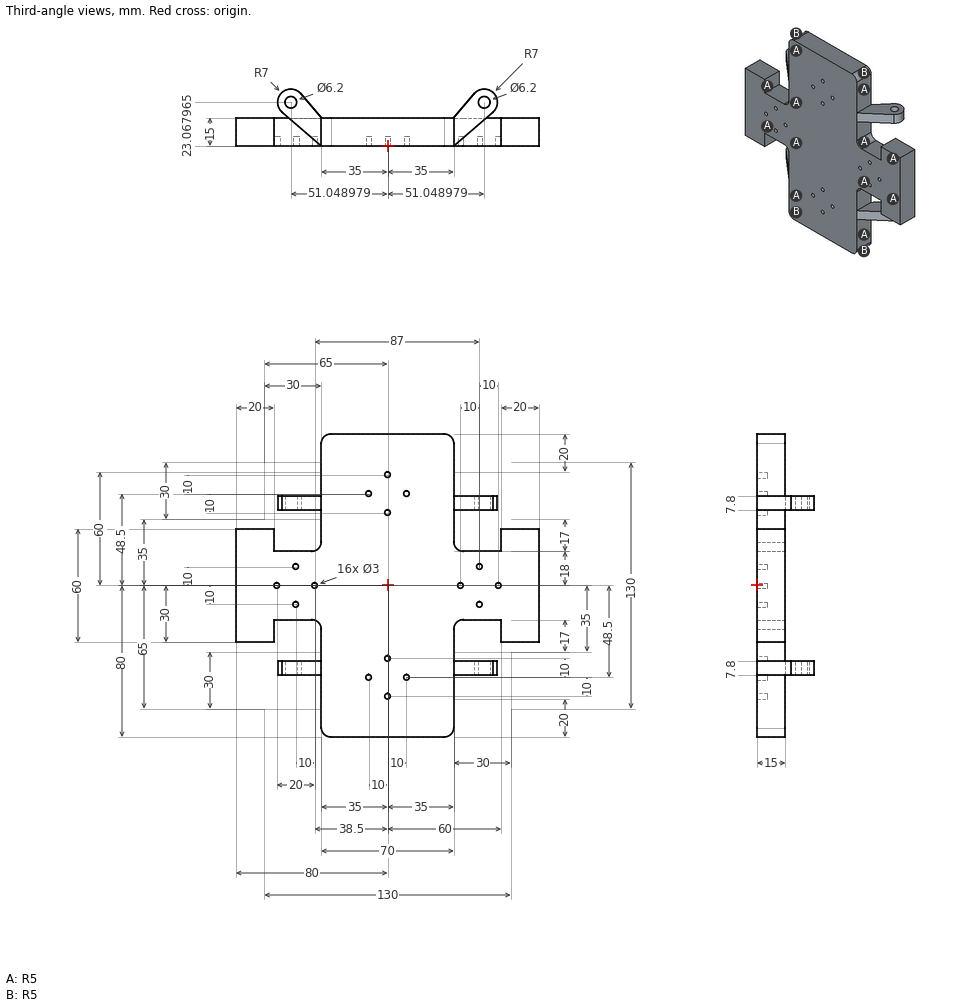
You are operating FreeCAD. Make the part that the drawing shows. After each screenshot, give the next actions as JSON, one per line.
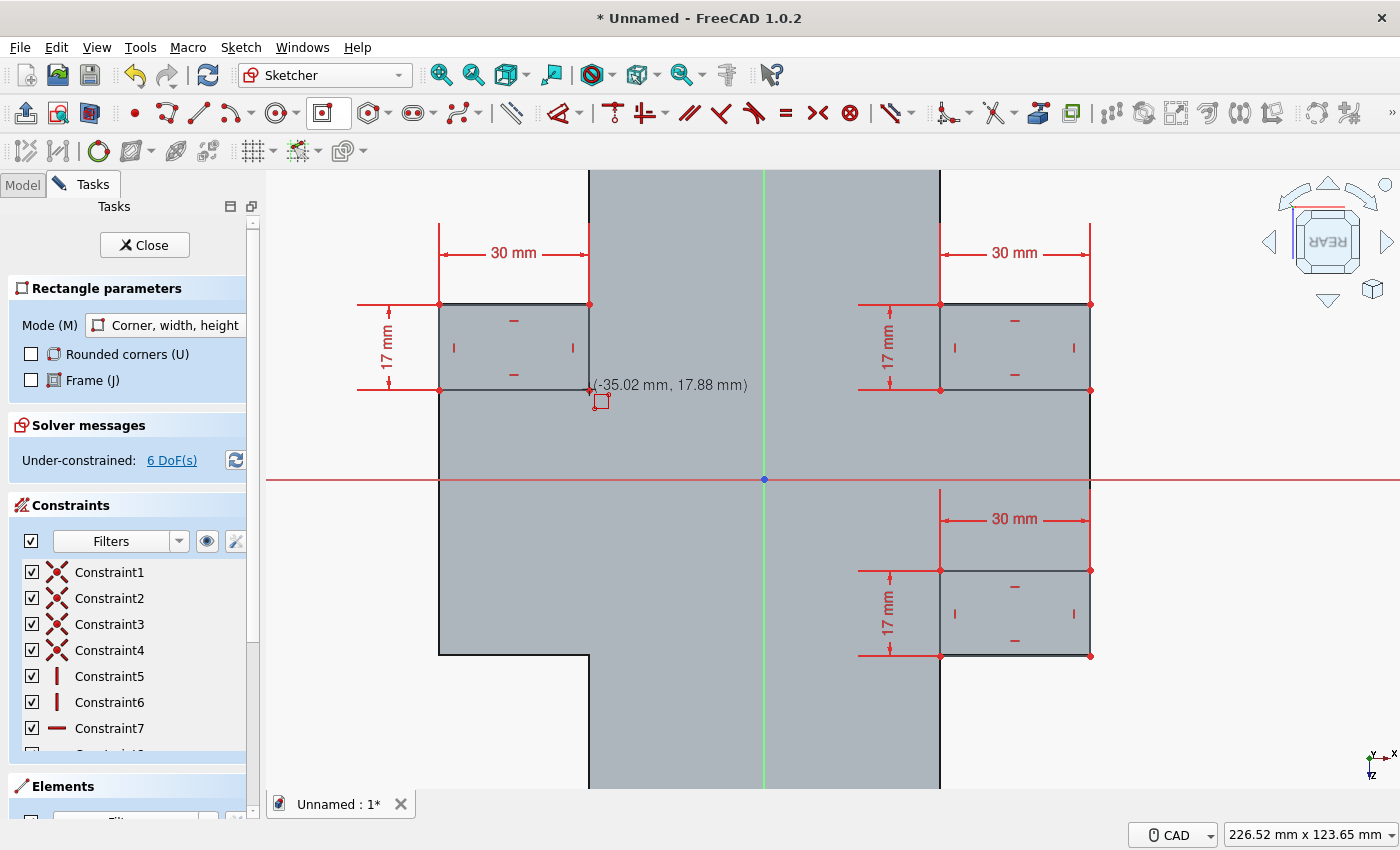
{"action": "left_click", "coordinate": [439, 570]}
{"action": "mouse_move", "coordinate": [589, 655]}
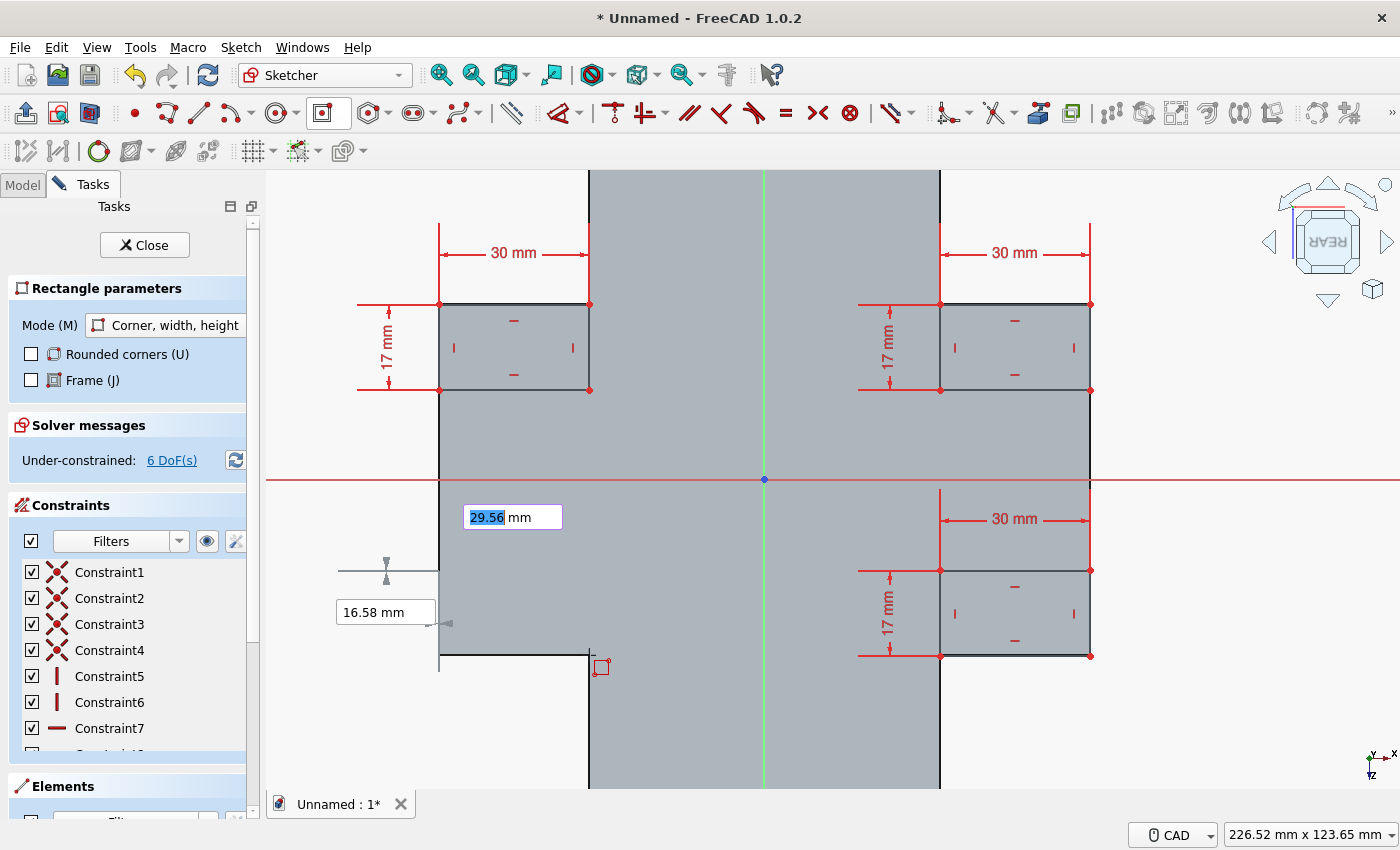
{"action": "type", "text": "30"}
{"action": "key", "text": "Tab"}
{"action": "type", "text": "17"}
{"action": "key", "text": "Return"}
{"action": "key", "text": "Escape"}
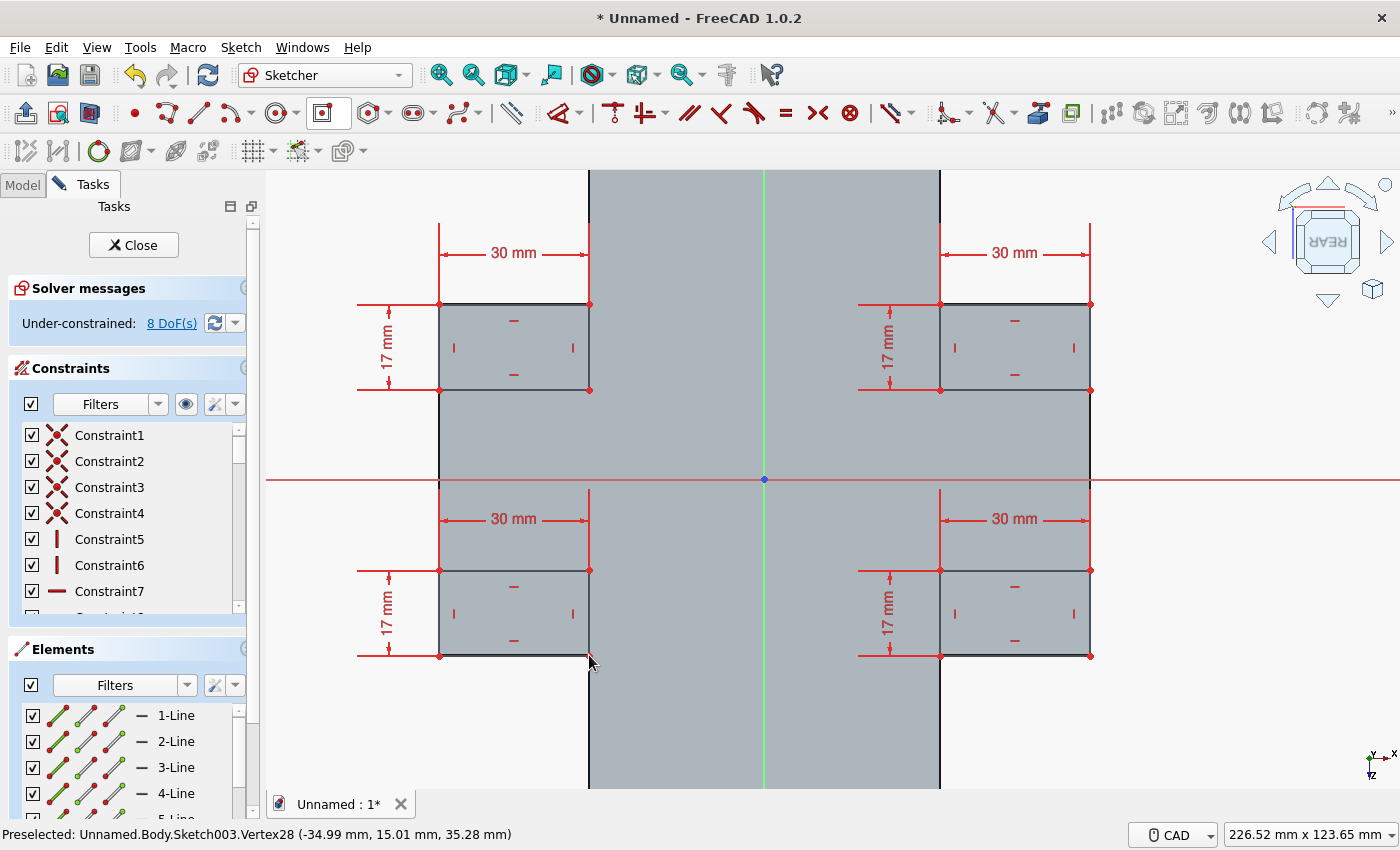
{"action": "left_click", "coordinate": [558, 114]}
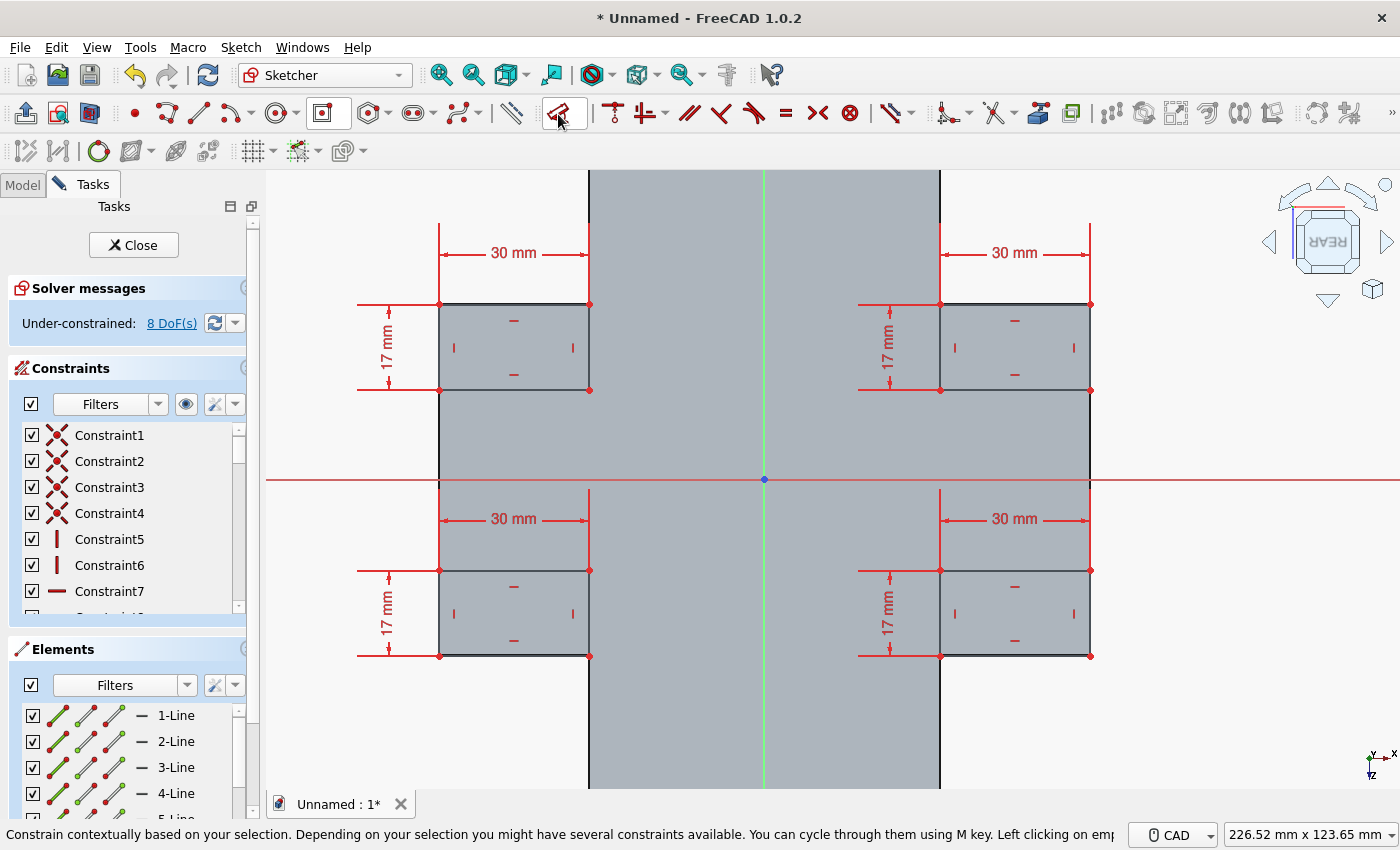
{"action": "left_click", "coordinate": [940, 305]}
{"action": "left_click", "coordinate": [852, 271]}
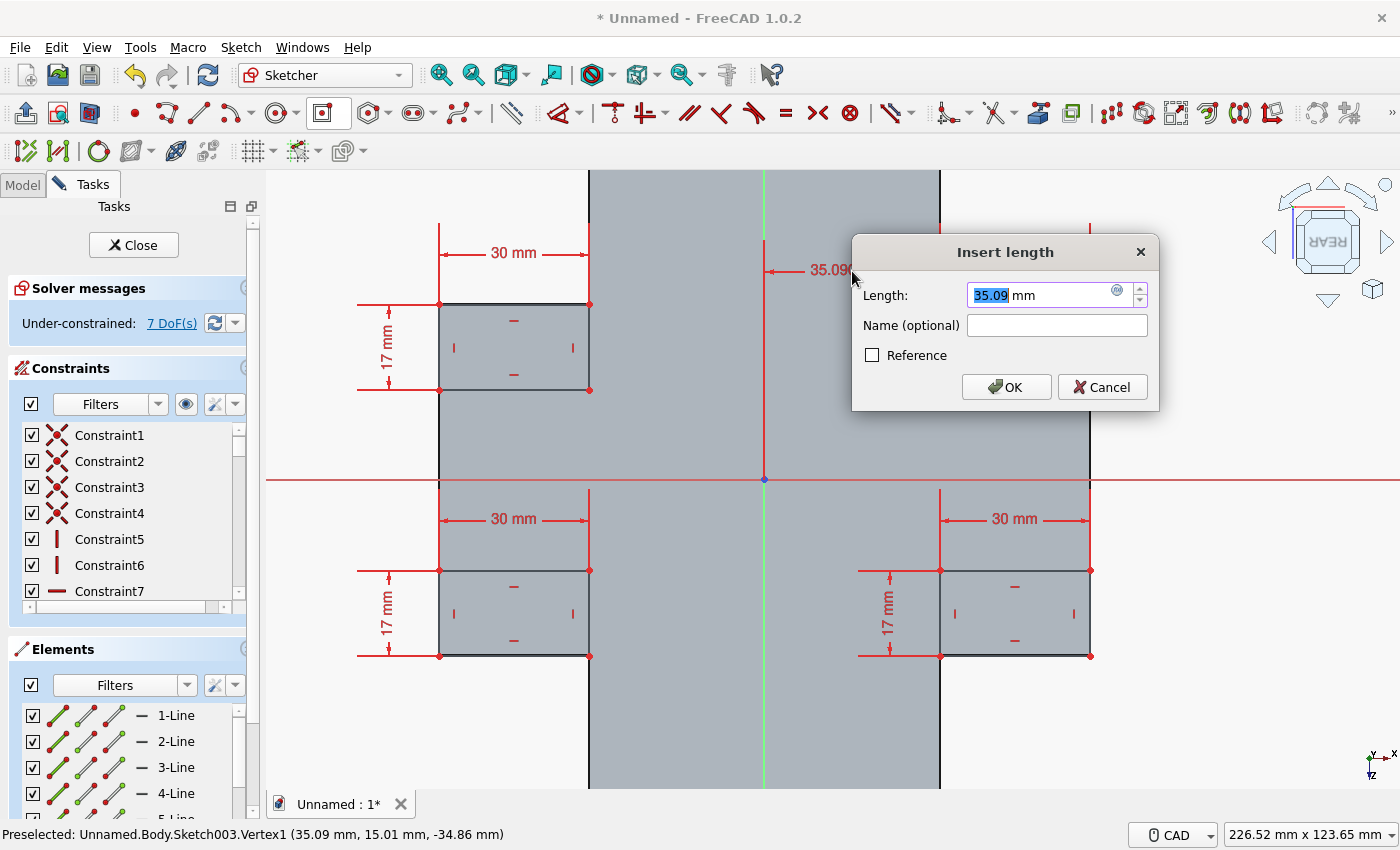
{"action": "type", "text": "35"}
{"action": "key", "text": "Return"}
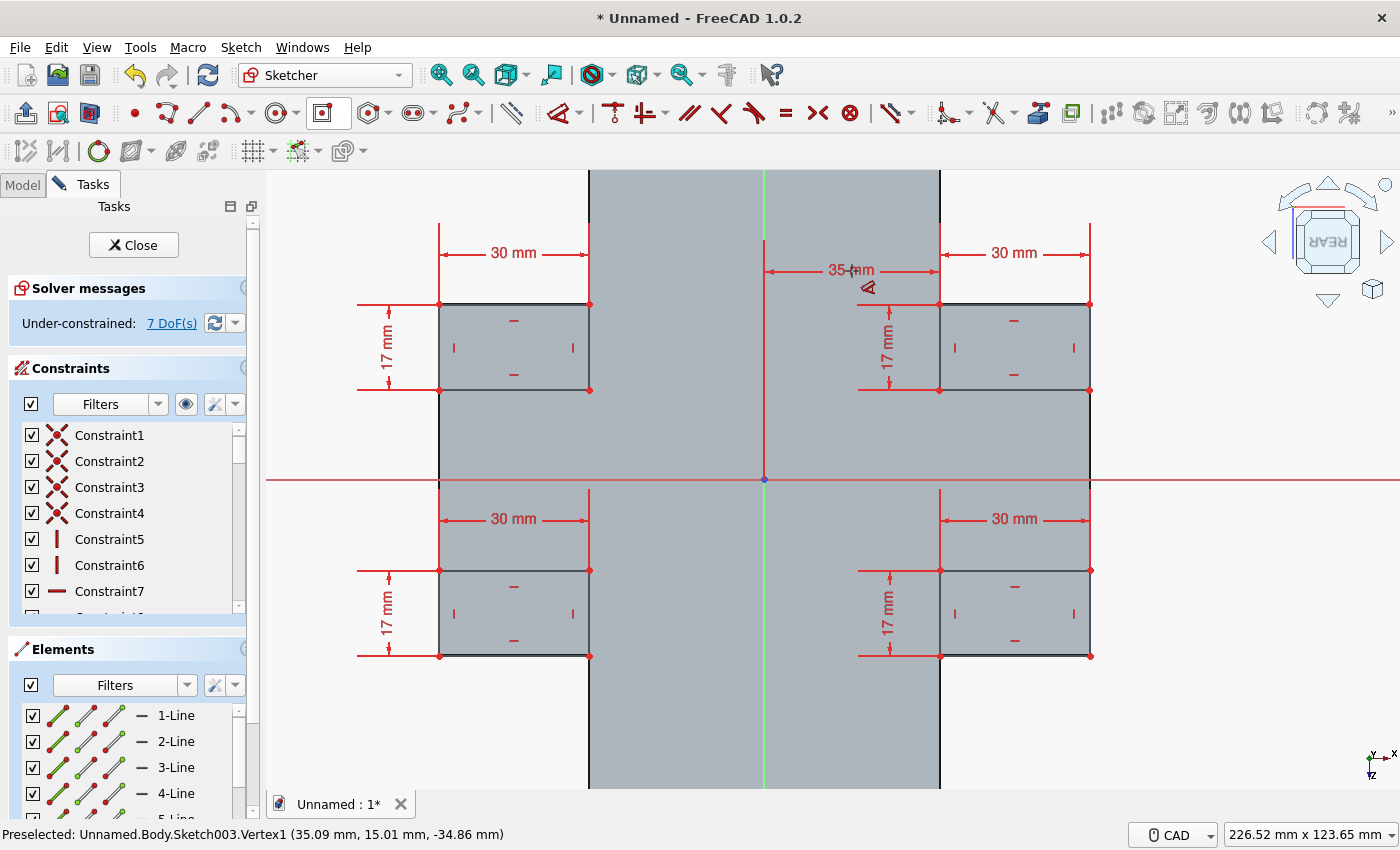
{"action": "left_click", "coordinate": [940, 305]}
{"action": "left_click", "coordinate": [974, 352]}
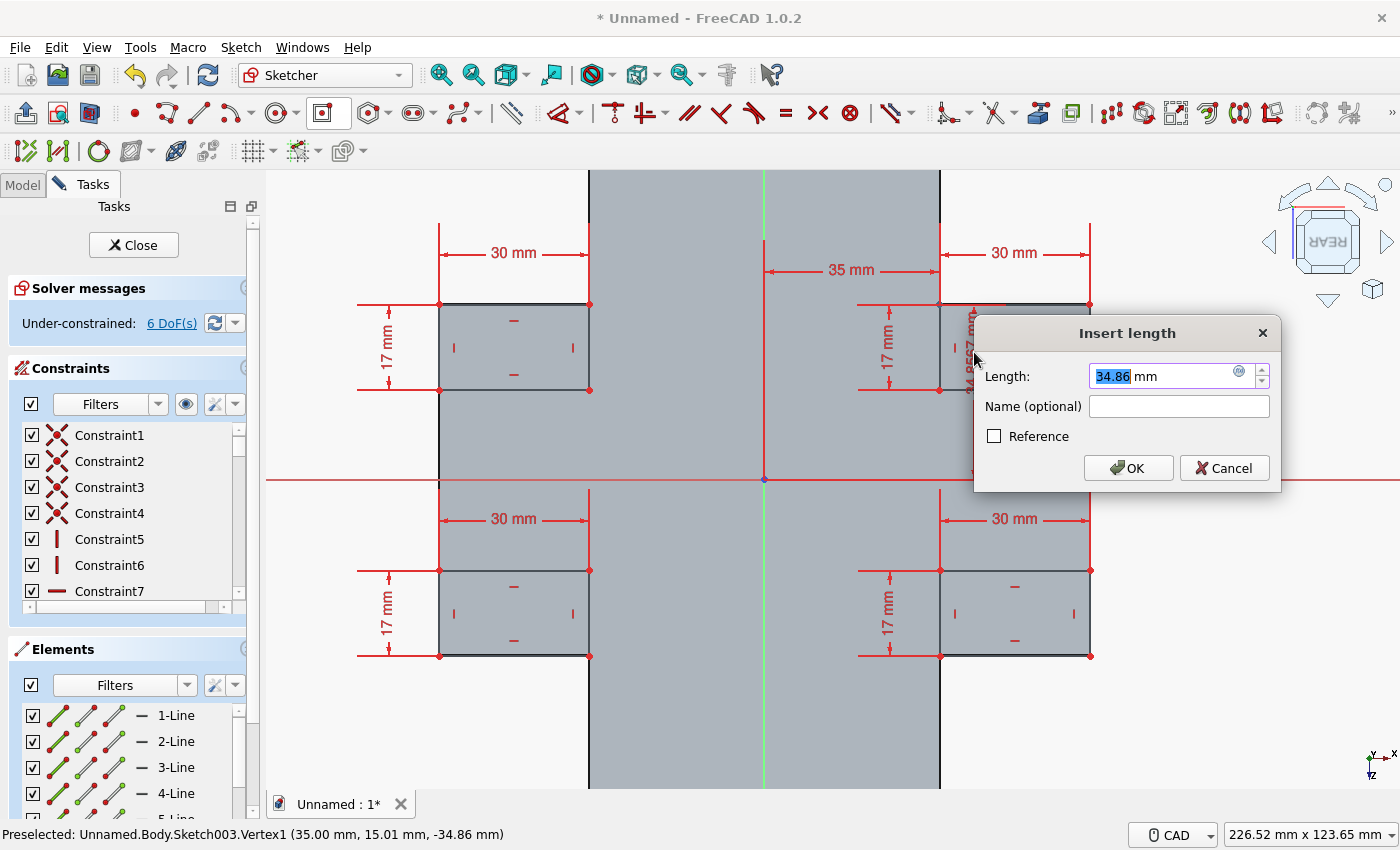
{"action": "type", "text": "35"}
{"action": "key", "text": "Return"}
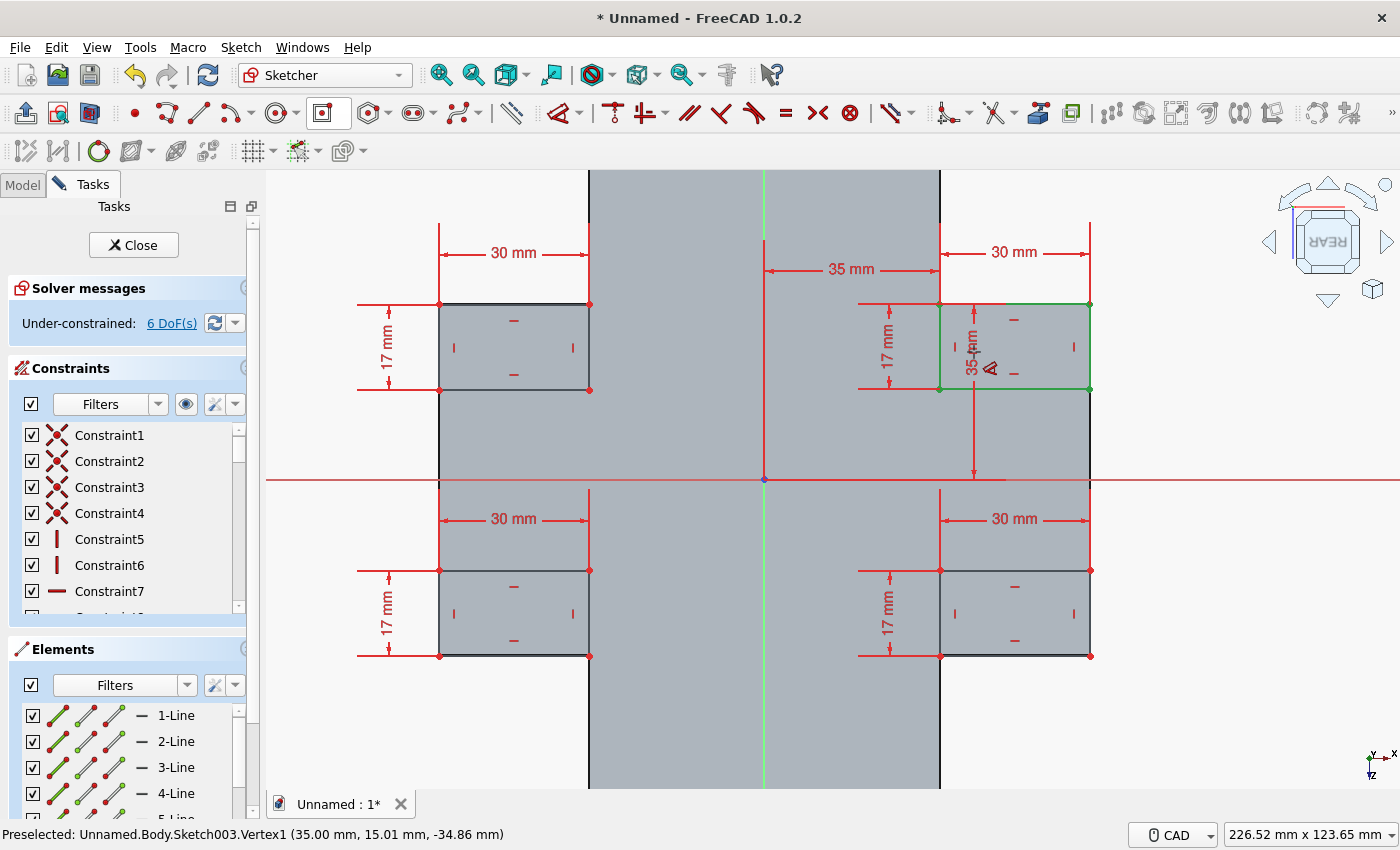
{"action": "left_click", "coordinate": [940, 571]}
{"action": "left_click", "coordinate": [852, 605]}